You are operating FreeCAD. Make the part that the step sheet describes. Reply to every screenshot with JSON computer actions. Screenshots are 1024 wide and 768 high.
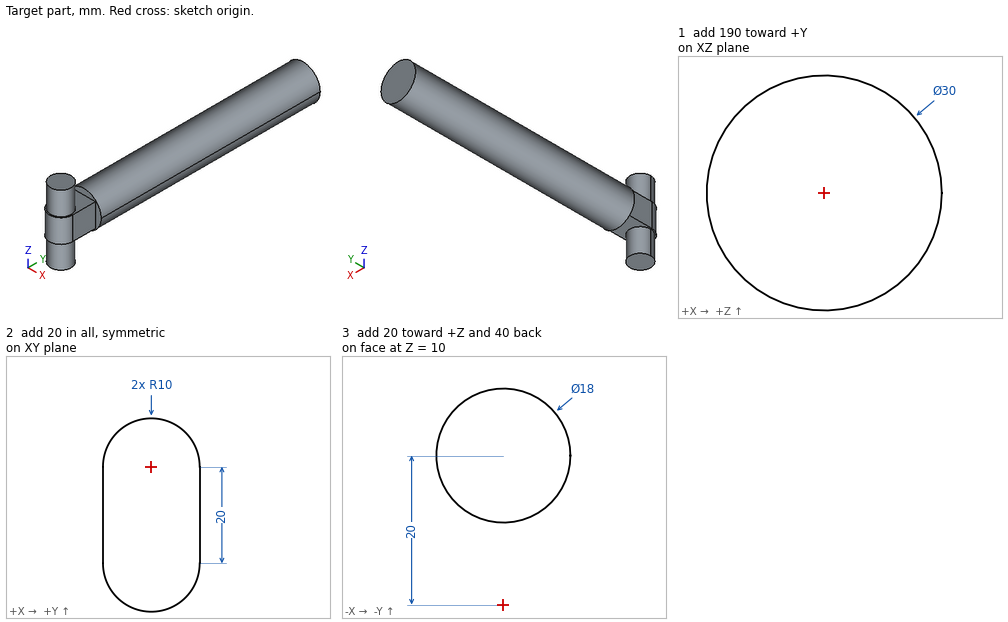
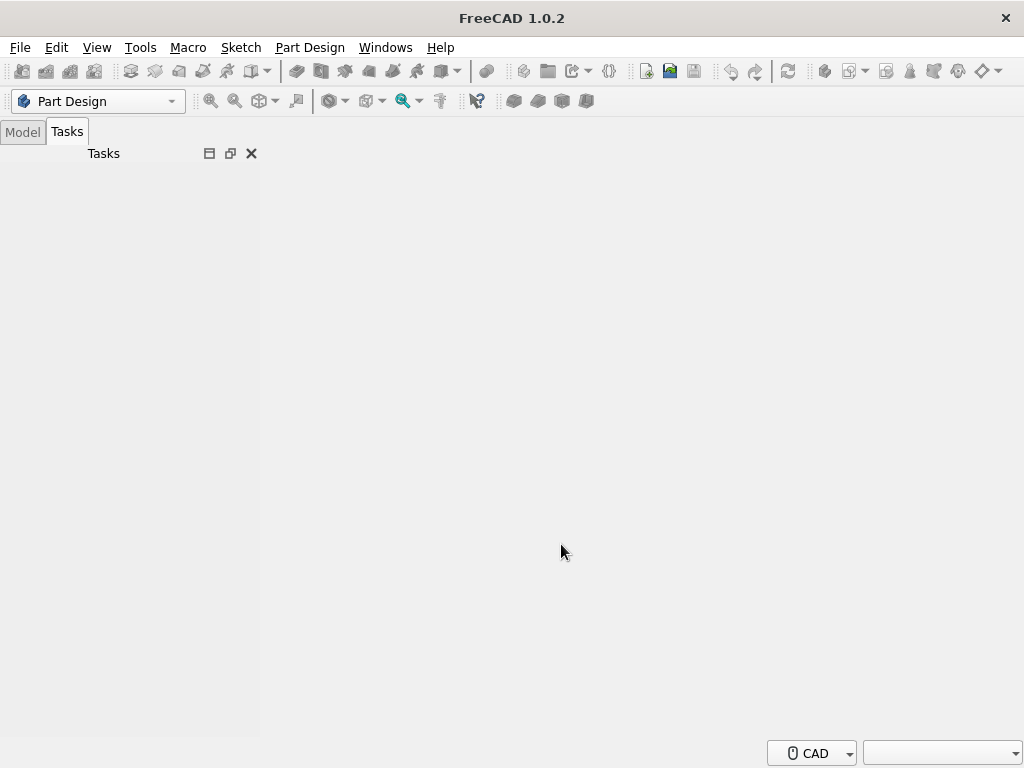
{"action": "left_click", "coordinate": [646, 72]}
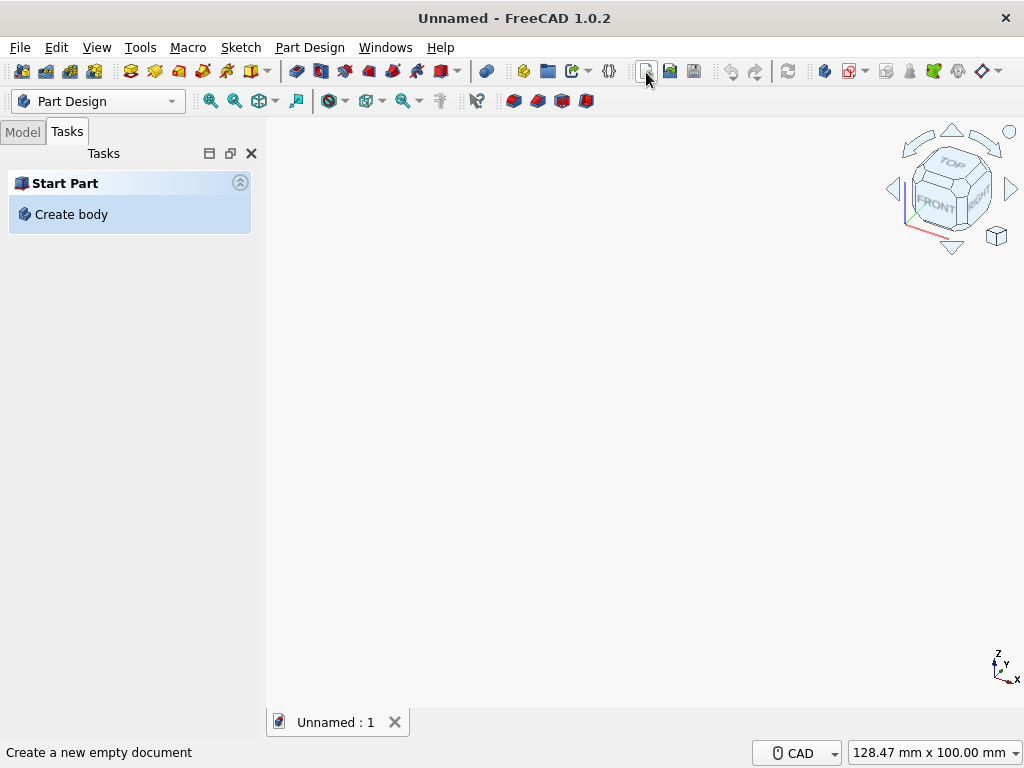
{"action": "left_click", "coordinate": [850, 72]}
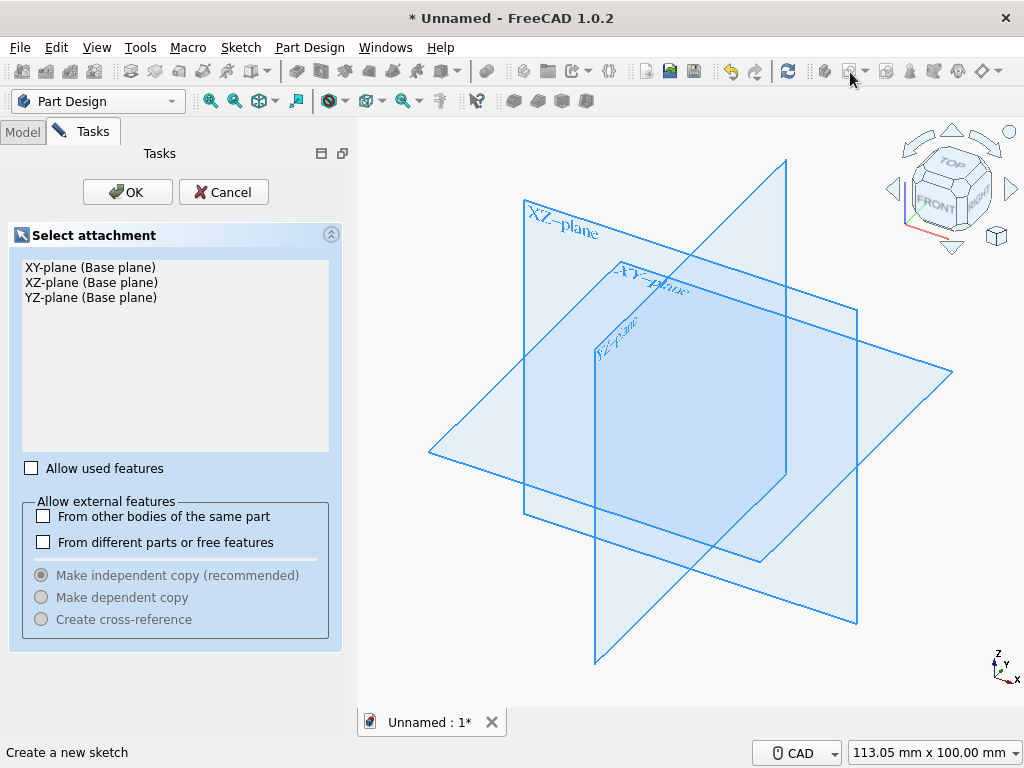
{"action": "left_click", "coordinate": [82, 282]}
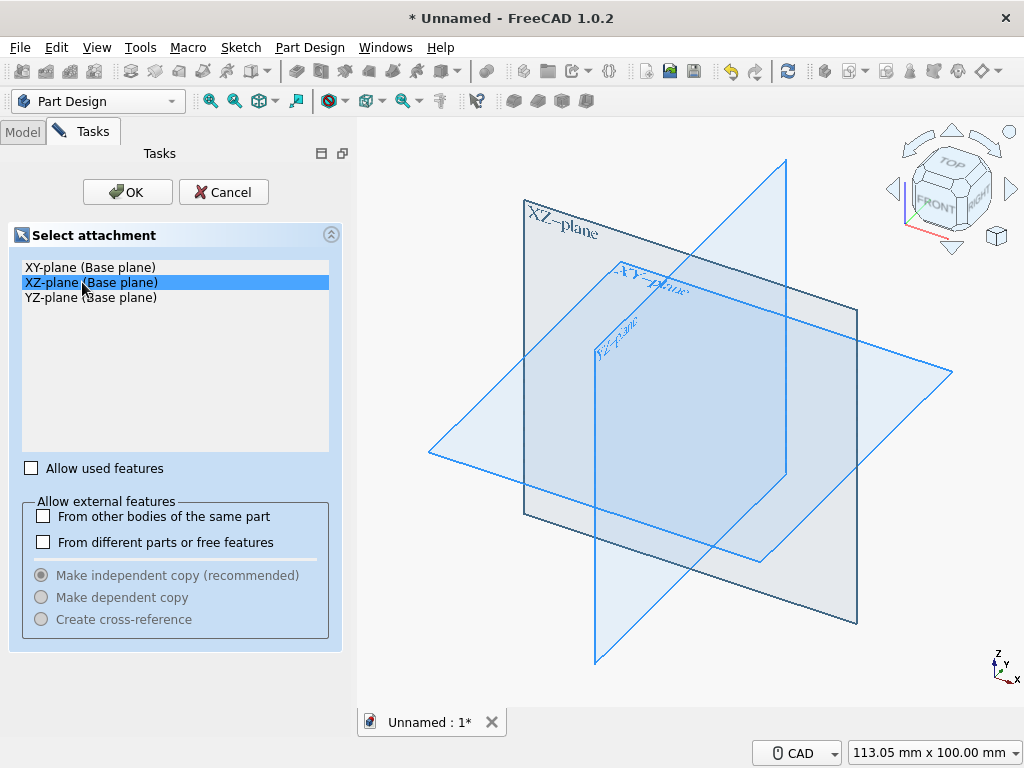
{"action": "left_click", "coordinate": [128, 192]}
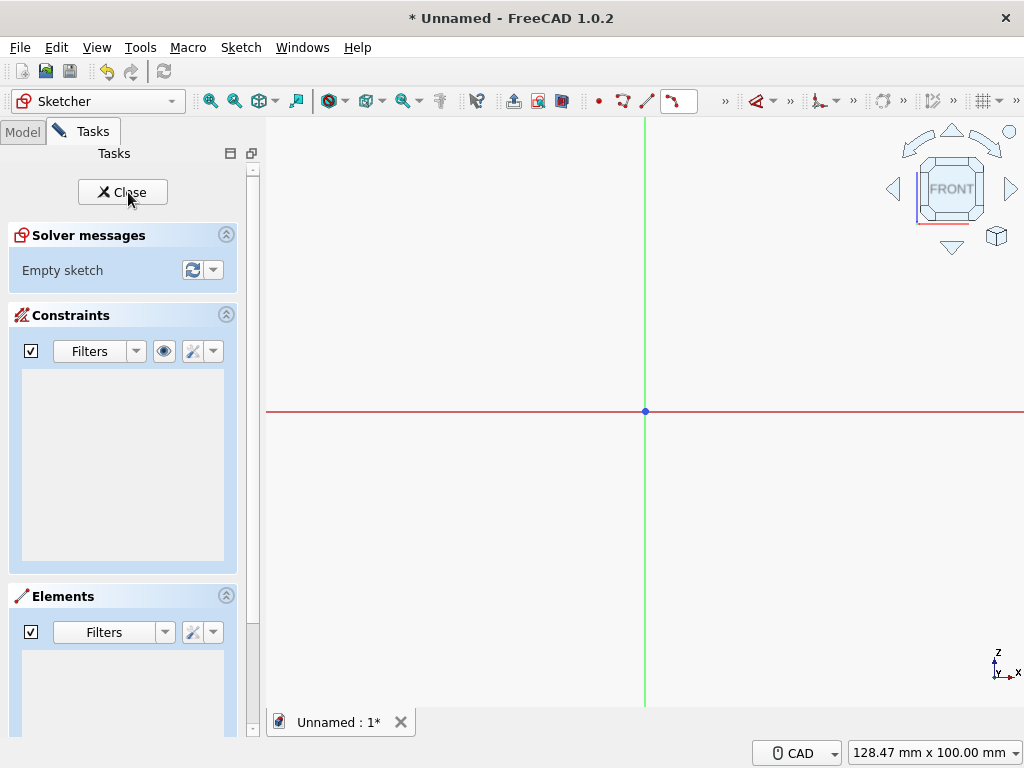
{"action": "scroll", "coordinate": [701, 412], "scroll_direction": "up", "scroll_amount": 4}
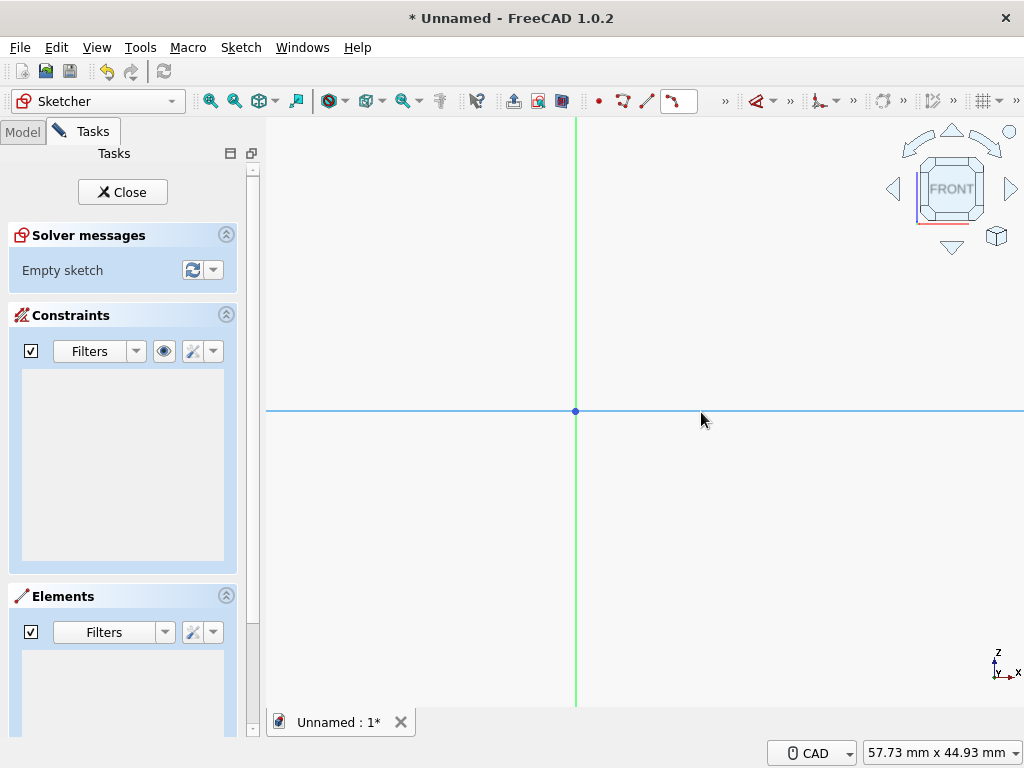
{"action": "key", "text": "g c"}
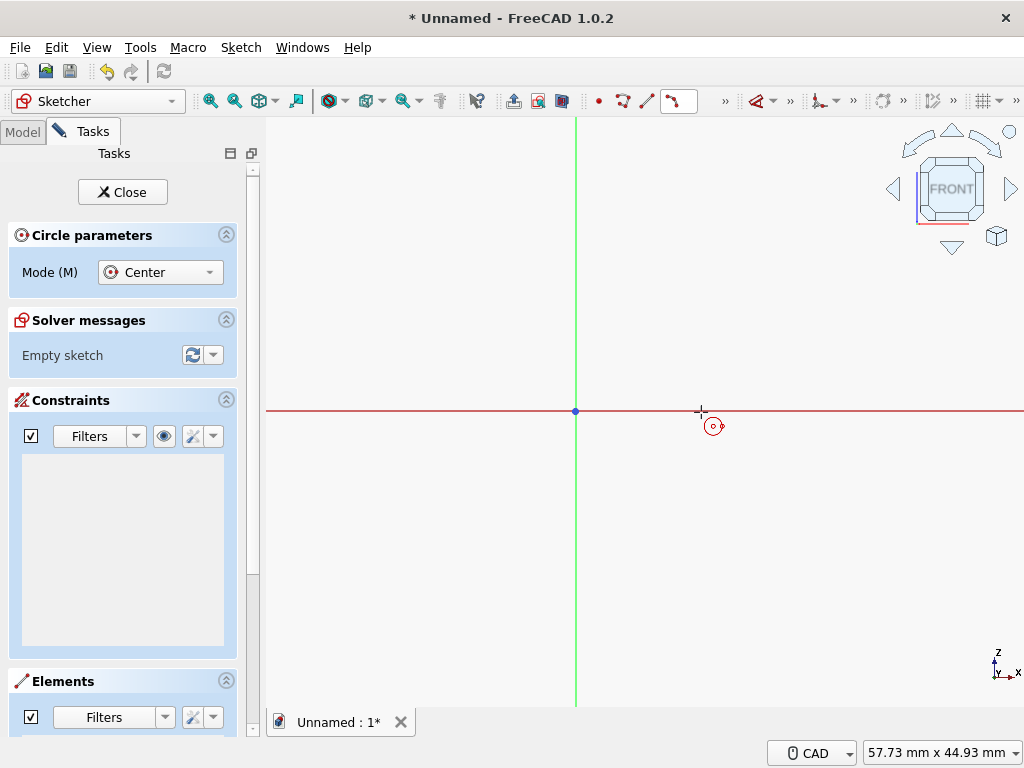
{"action": "left_click", "coordinate": [576, 411]}
{"action": "mouse_move", "coordinate": [715, 272]}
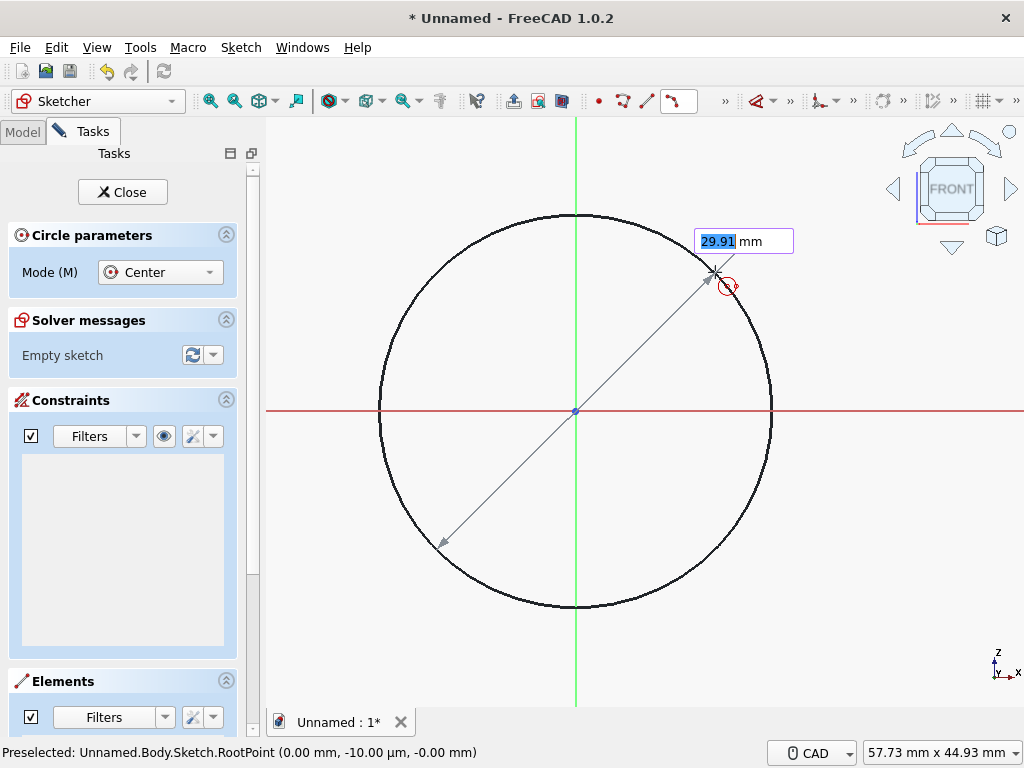
{"action": "type", "text": "30"}
{"action": "key", "text": "Return"}
{"action": "key", "text": "Escape"}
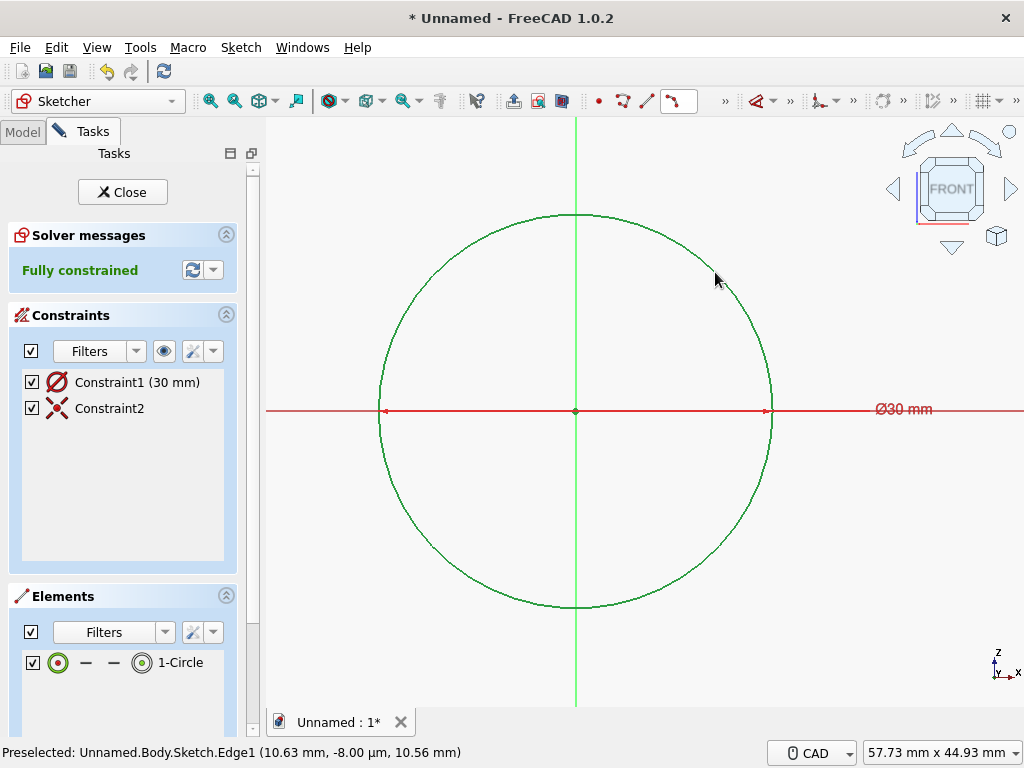
{"action": "left_click", "coordinate": [123, 192]}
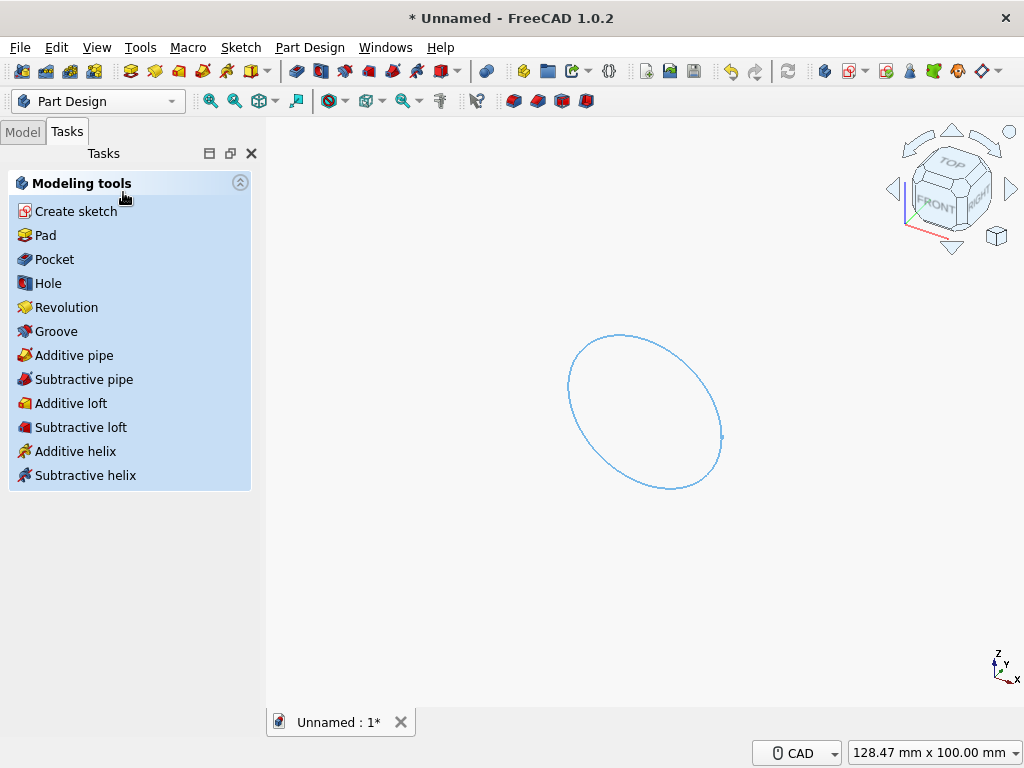
{"action": "left_click", "coordinate": [132, 72]}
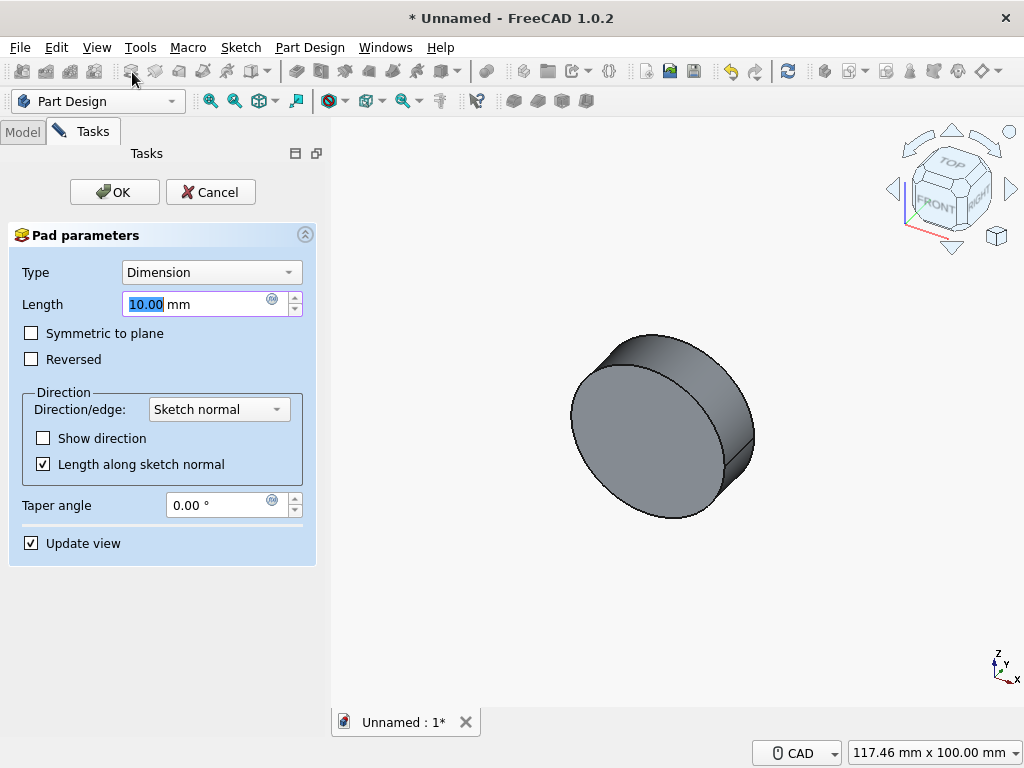
{"action": "type", "text": "190"}
{"action": "key", "text": "Tab"}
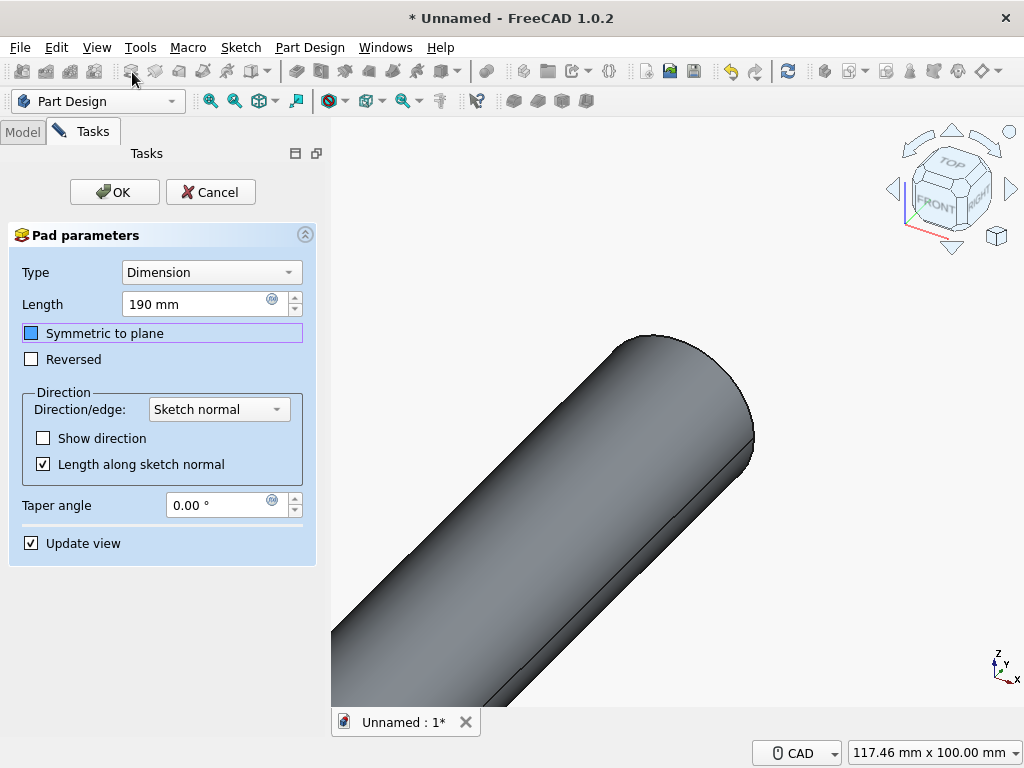
{"action": "left_click", "coordinate": [30, 359]}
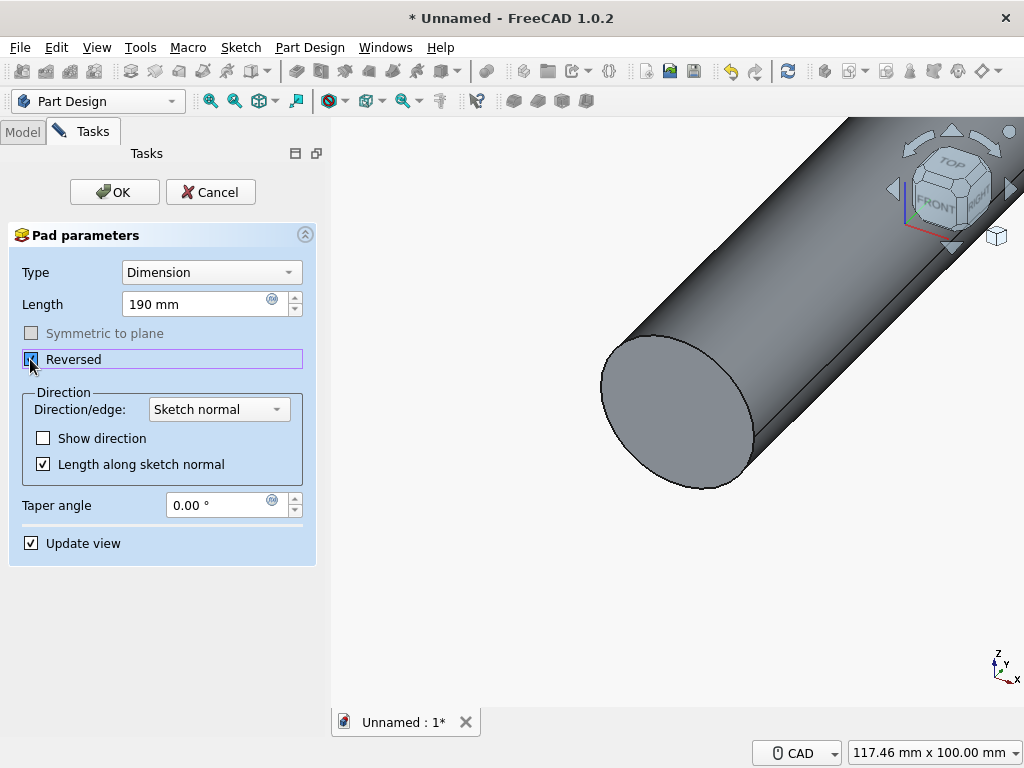
{"action": "left_click", "coordinate": [115, 192]}